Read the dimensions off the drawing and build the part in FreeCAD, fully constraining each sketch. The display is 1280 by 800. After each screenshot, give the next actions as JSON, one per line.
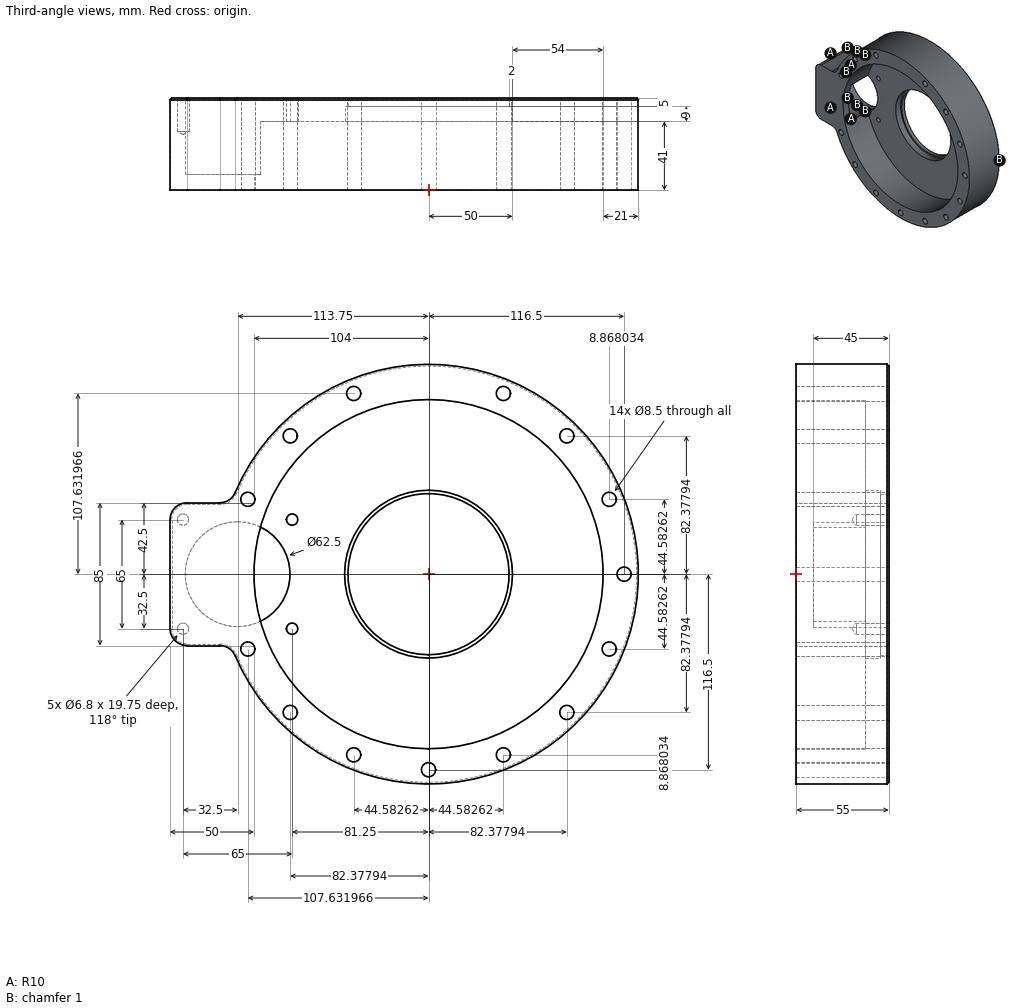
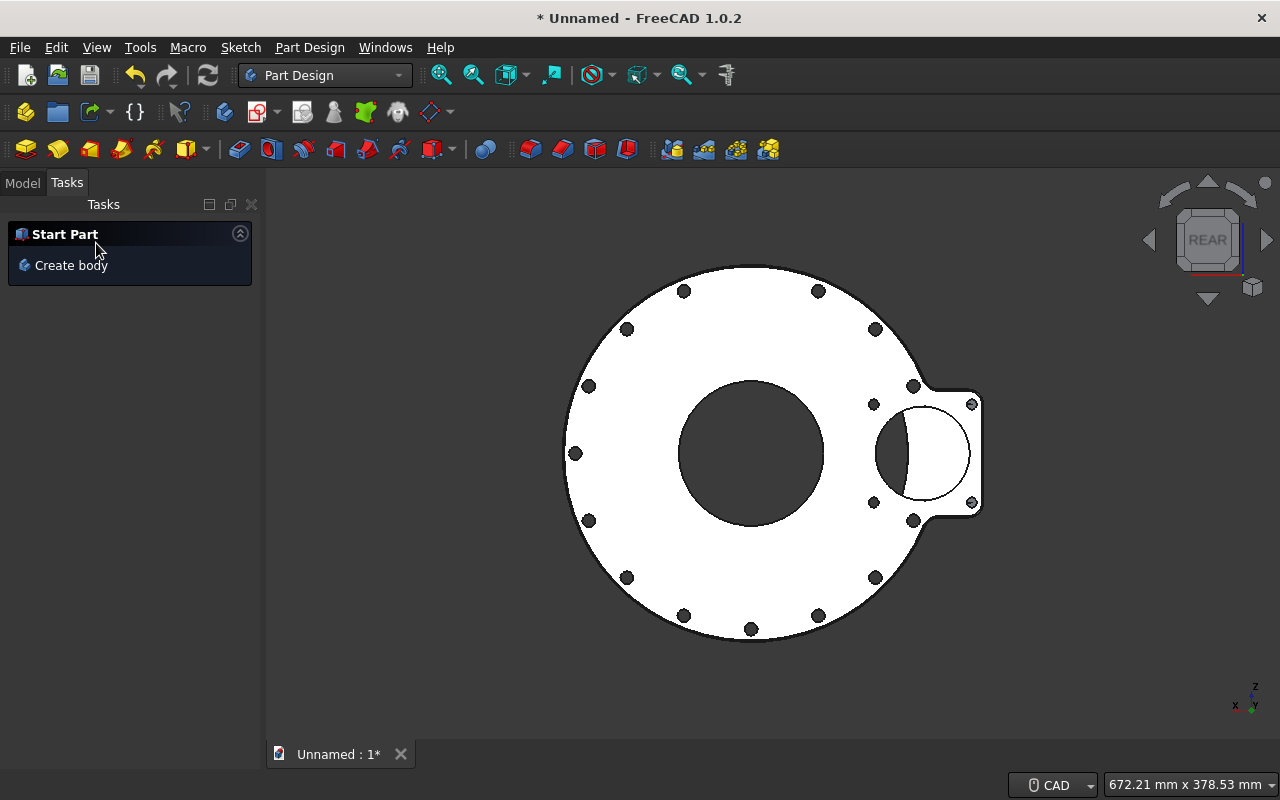
{"action": "key", "text": "0"}